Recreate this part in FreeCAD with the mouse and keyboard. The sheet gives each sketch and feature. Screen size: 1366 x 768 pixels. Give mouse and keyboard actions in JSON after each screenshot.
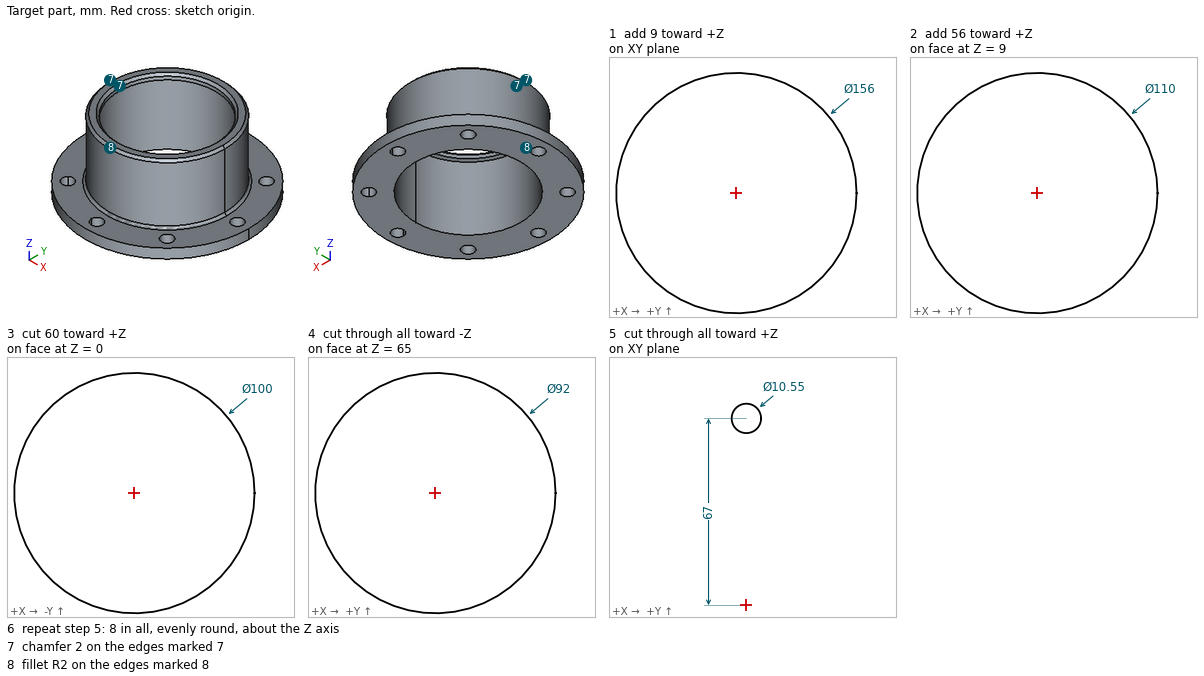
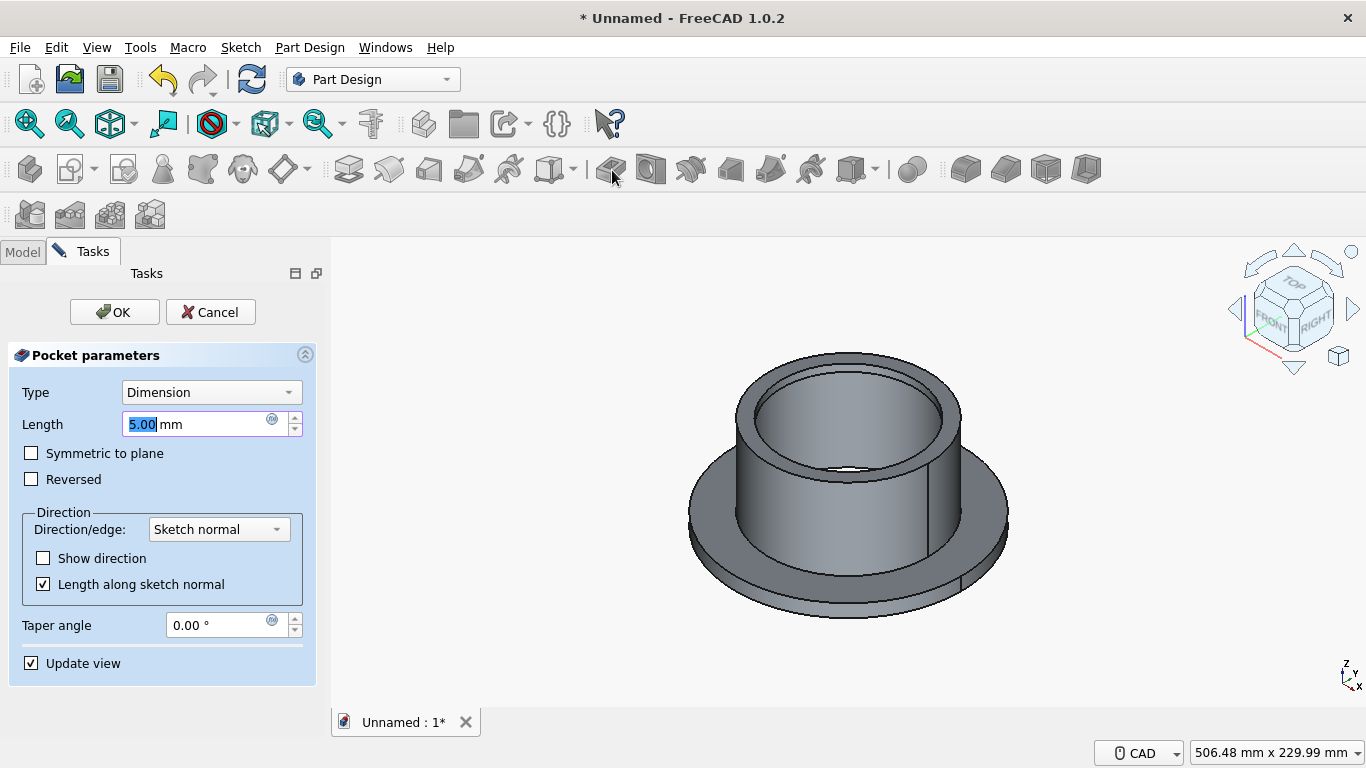
{"action": "left_click", "coordinate": [212, 392]}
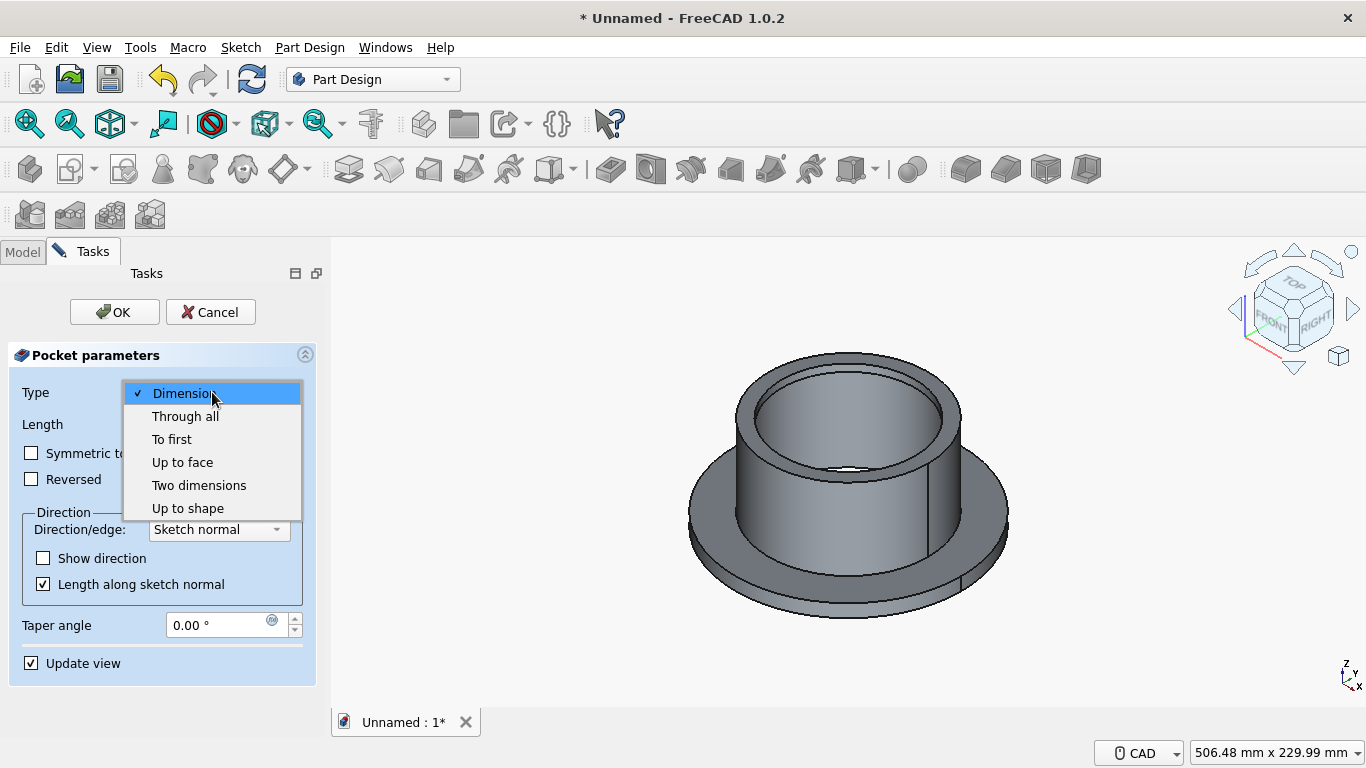
{"action": "left_click", "coordinate": [212, 416]}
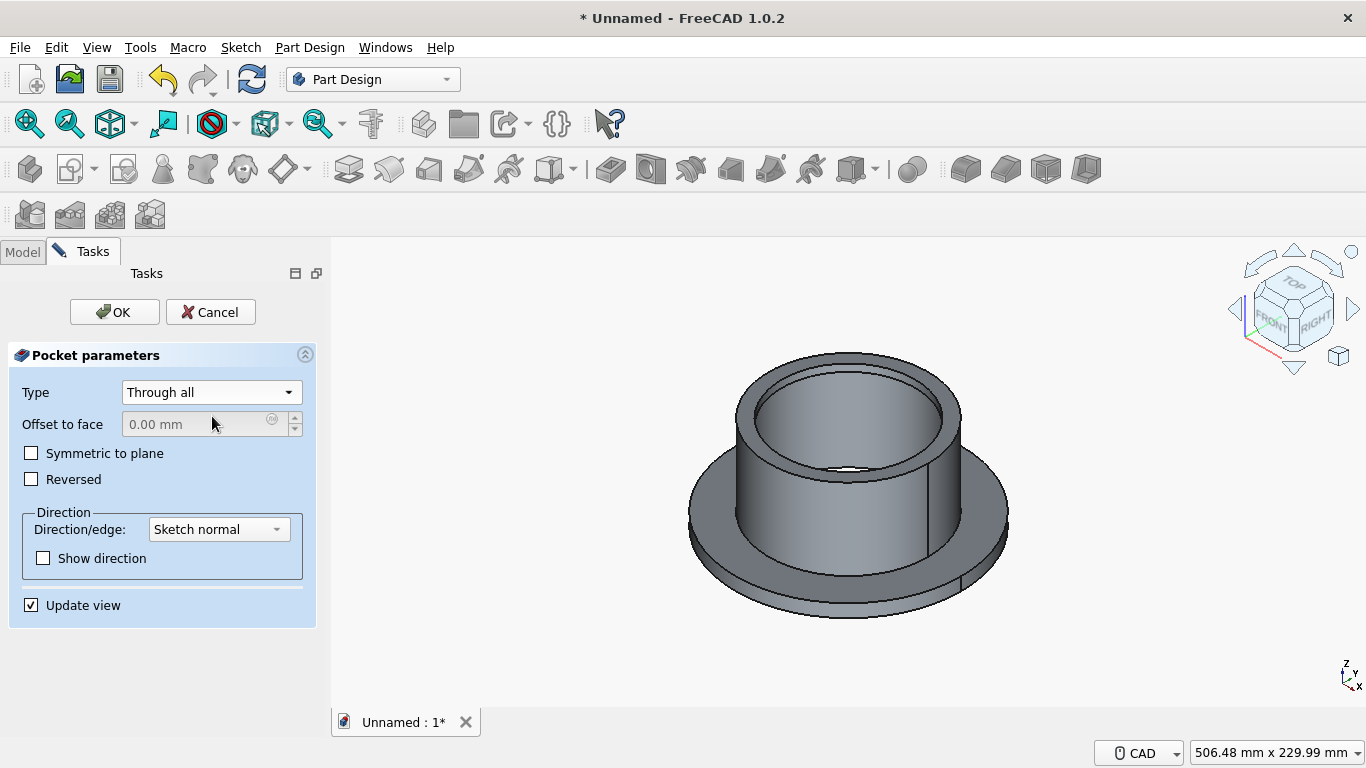
{"action": "left_click", "coordinate": [30, 479]}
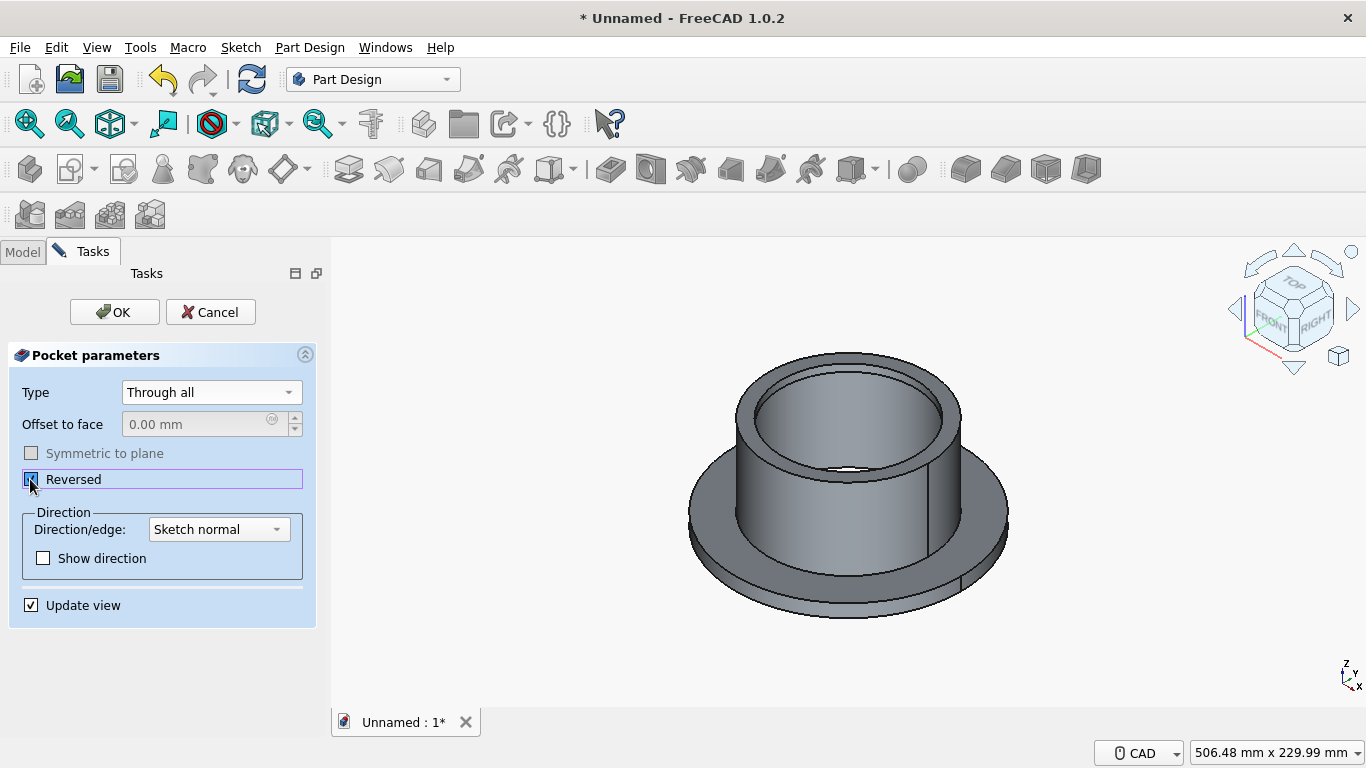
{"action": "left_click", "coordinate": [115, 312]}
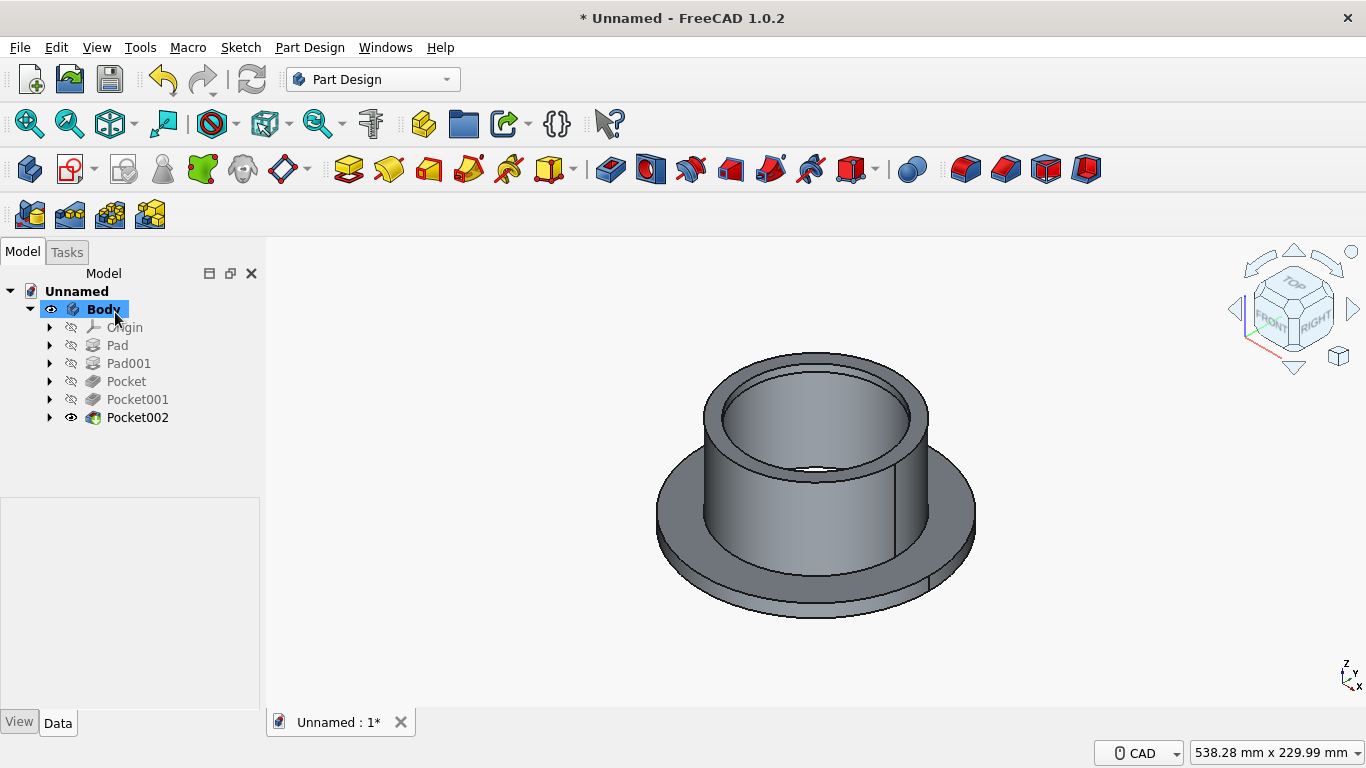
{"action": "left_click", "coordinate": [116, 417]}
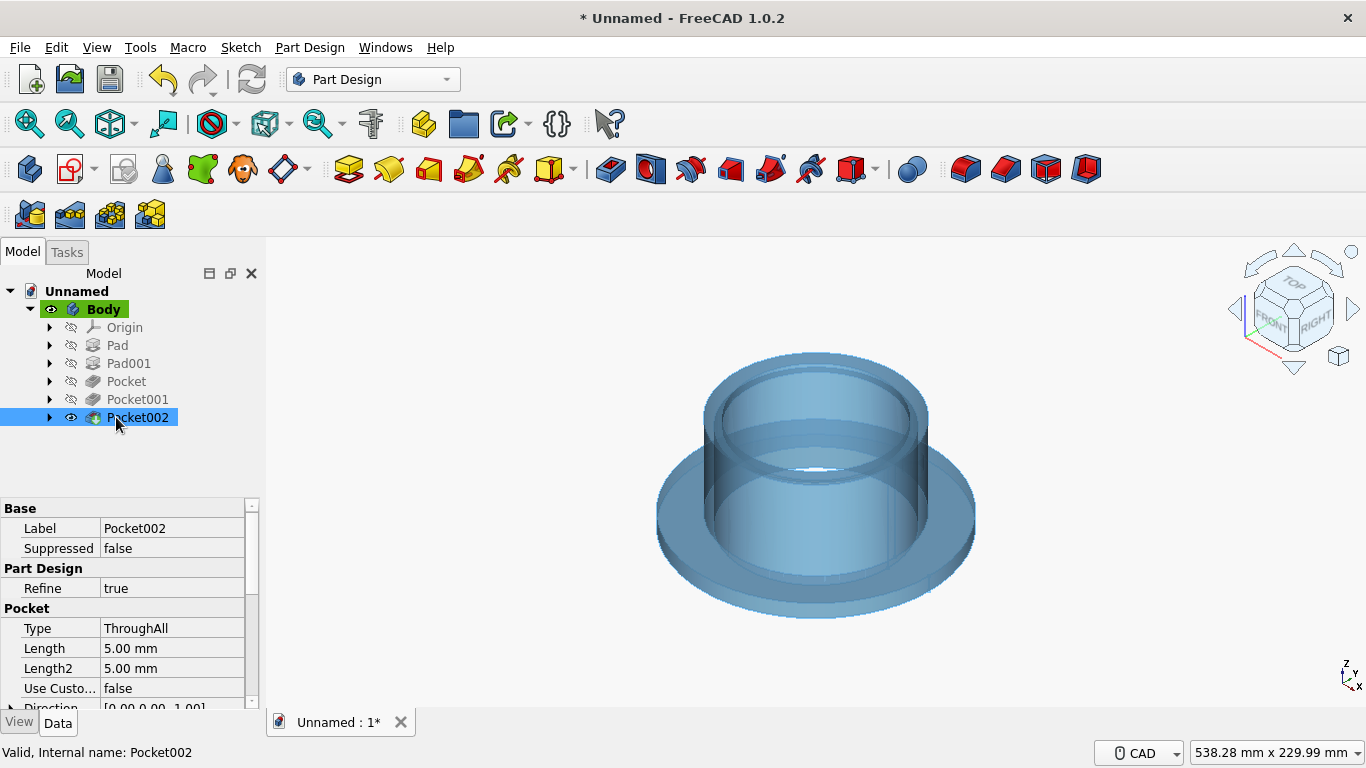
{"action": "left_click", "coordinate": [110, 214]}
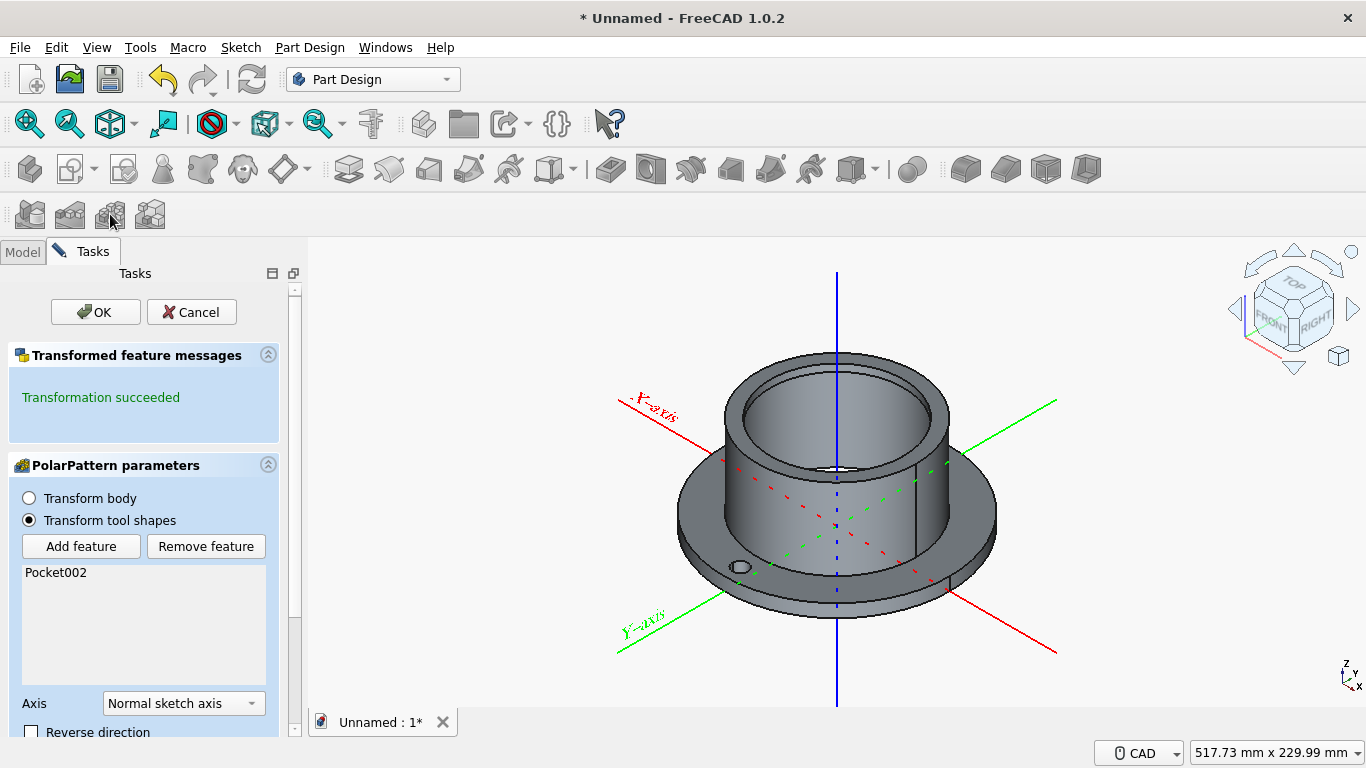
{"action": "left_click", "coordinate": [184, 704]}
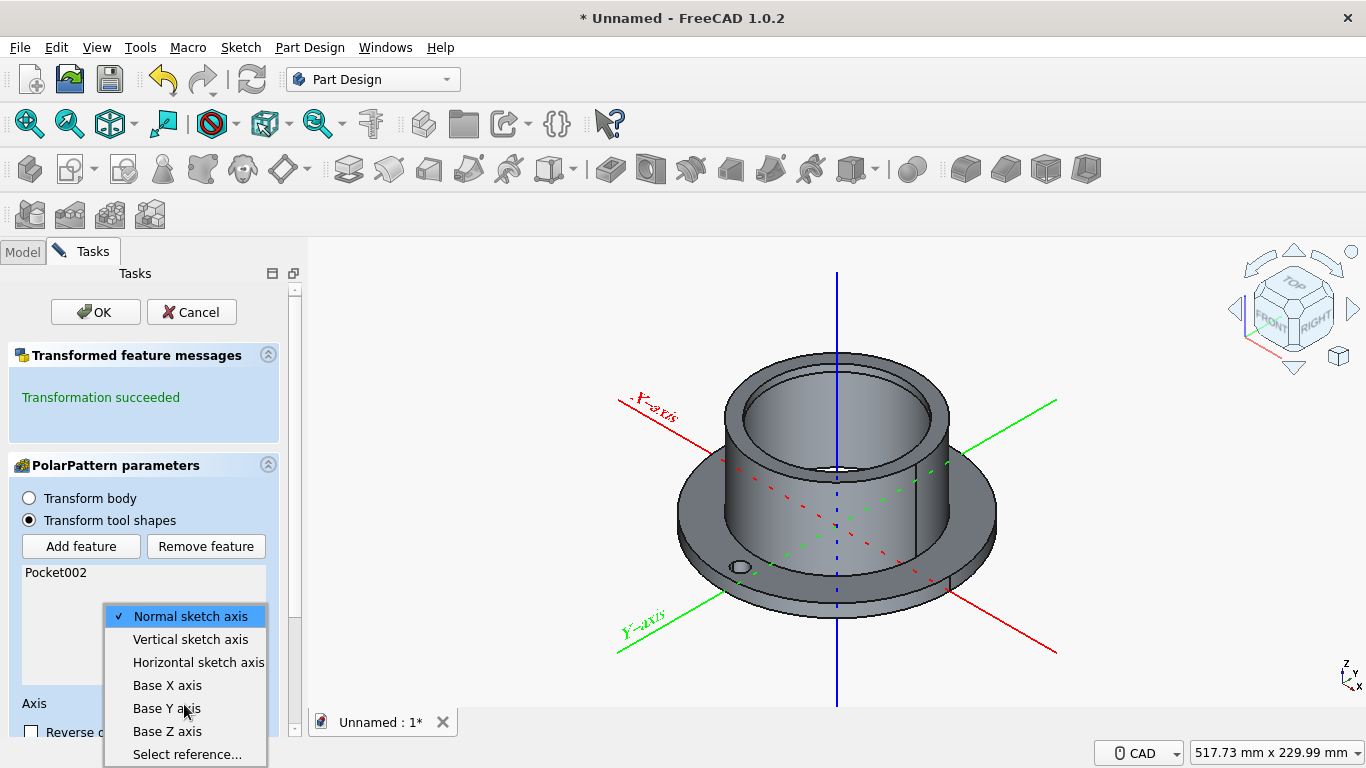
{"action": "left_click", "coordinate": [184, 732]}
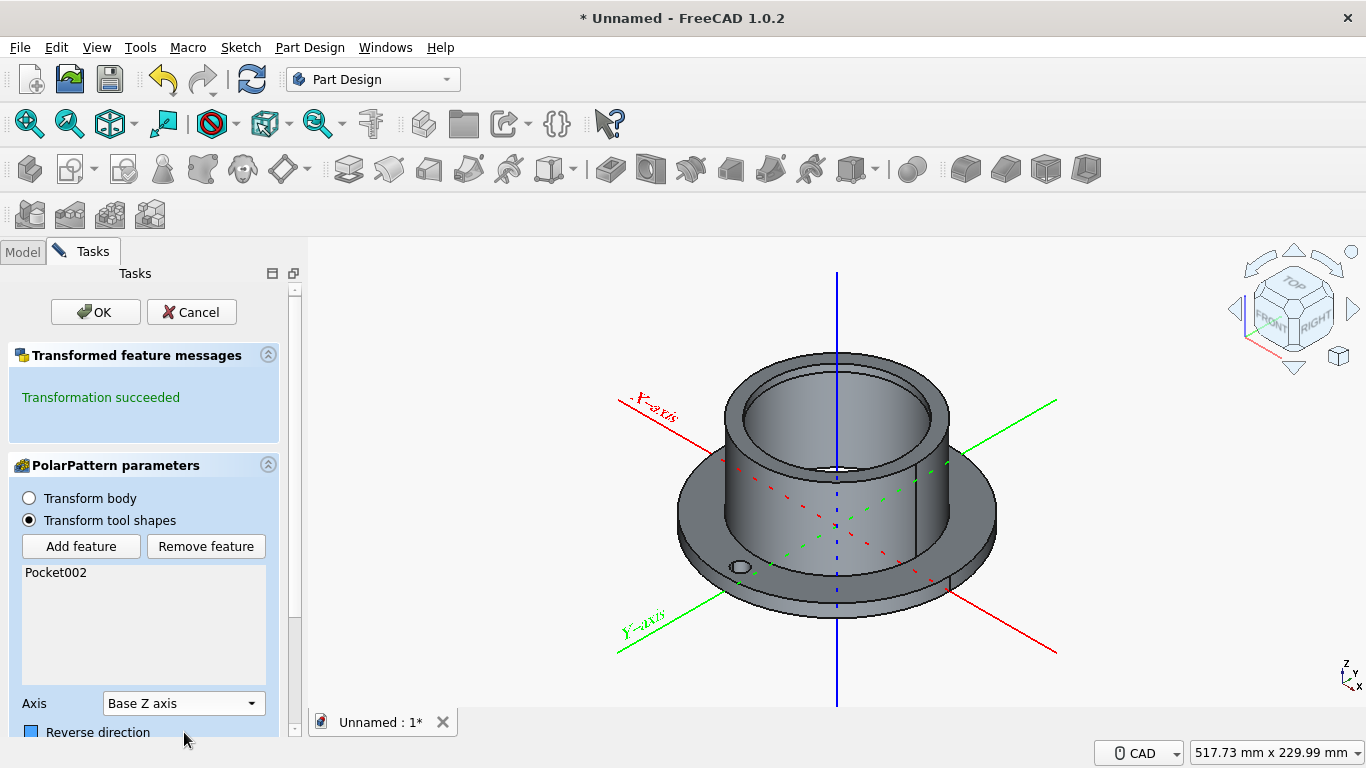
{"action": "scroll", "coordinate": [295, 510], "scroll_direction": "down", "scroll_amount": 3}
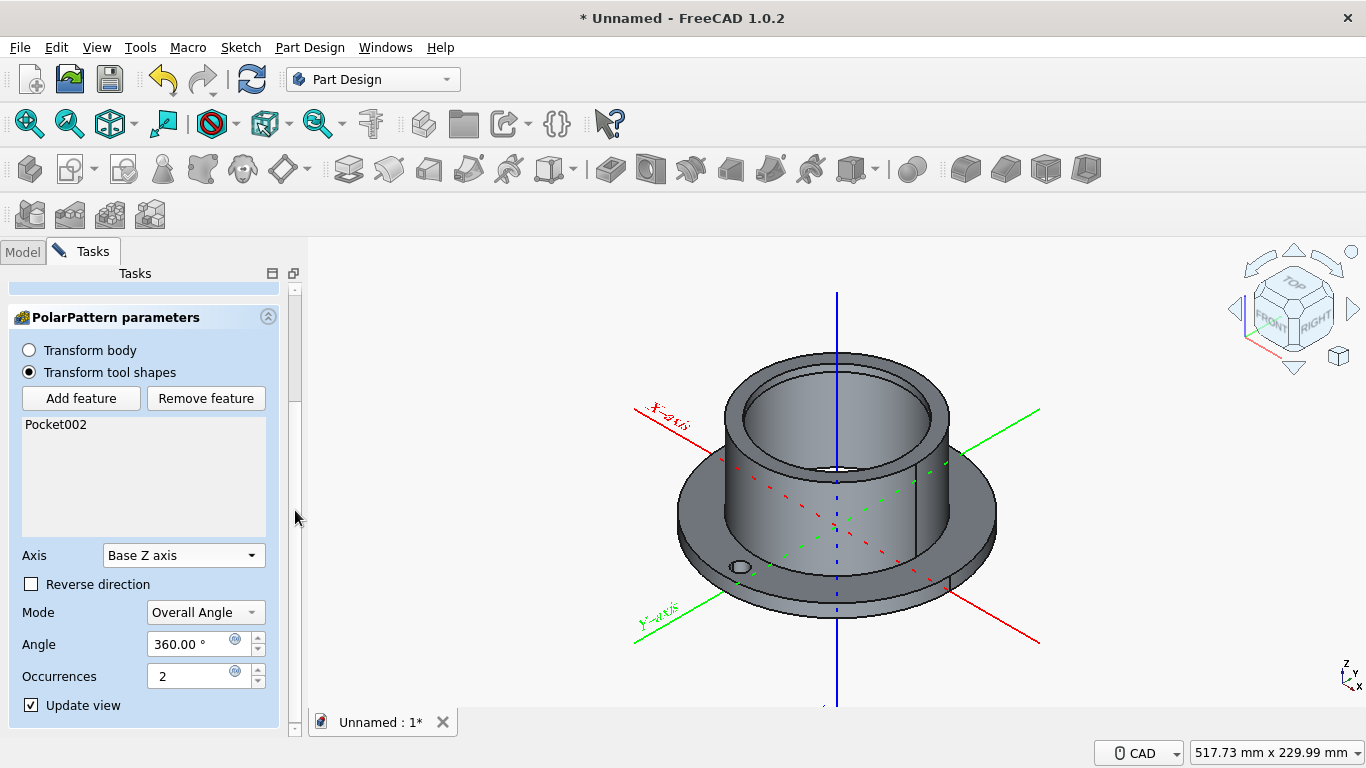
{"action": "triple_click", "coordinate": [198, 676]}